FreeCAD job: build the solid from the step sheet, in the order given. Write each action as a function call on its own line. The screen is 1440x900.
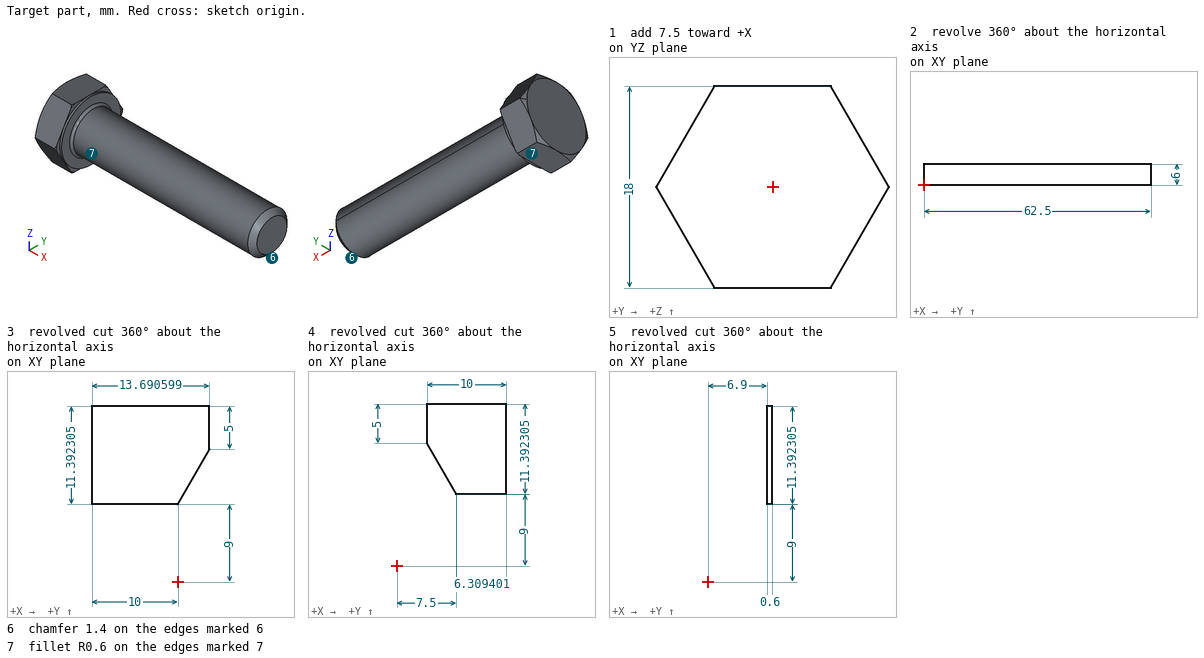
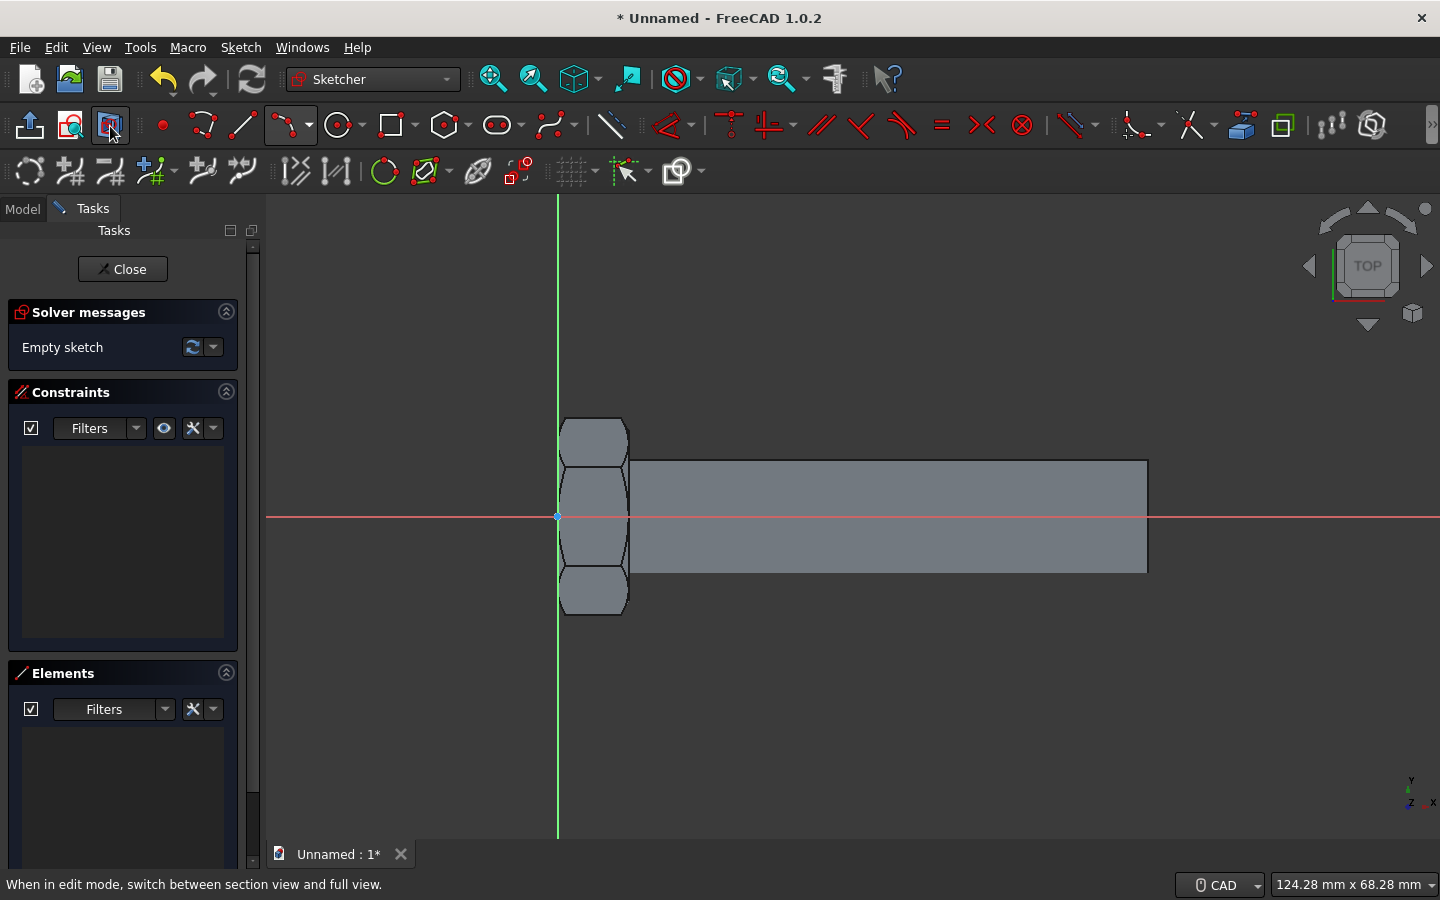
scroll(437, 342, up, 4)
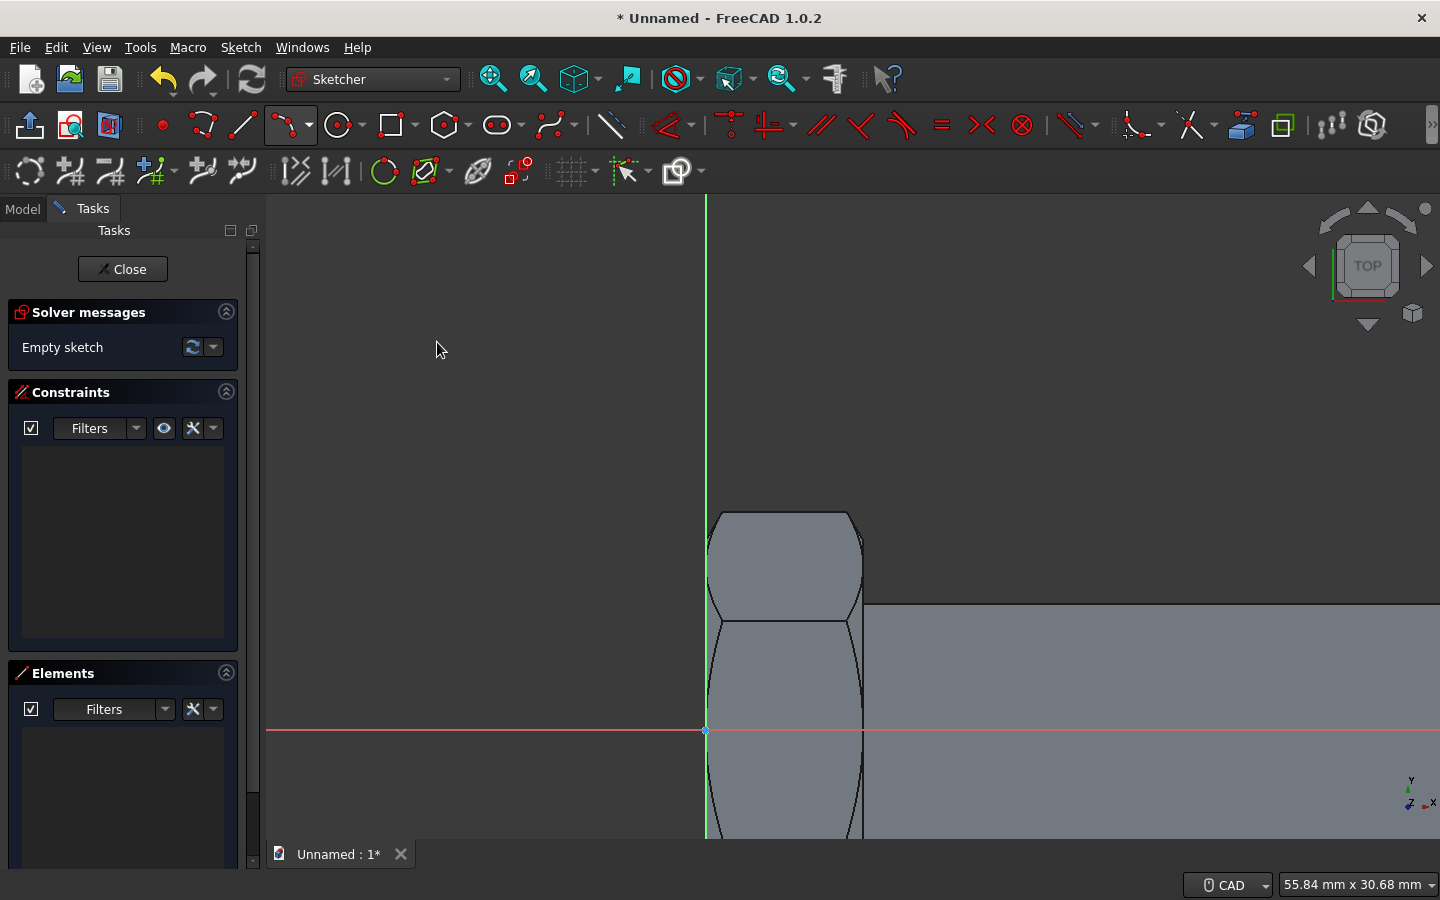
click(392, 126)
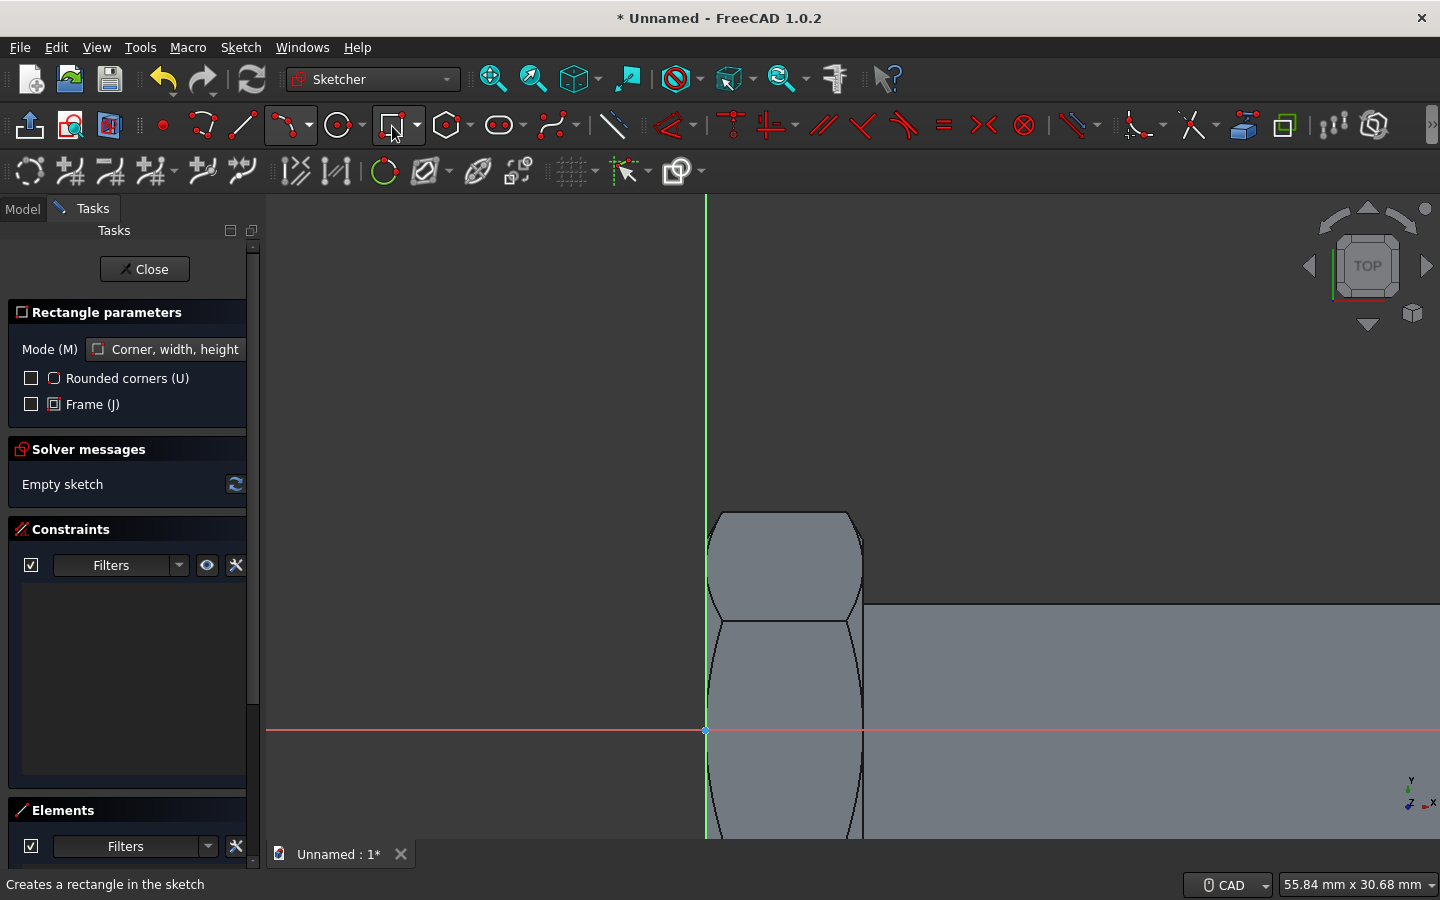
scroll(851, 301, up, 2)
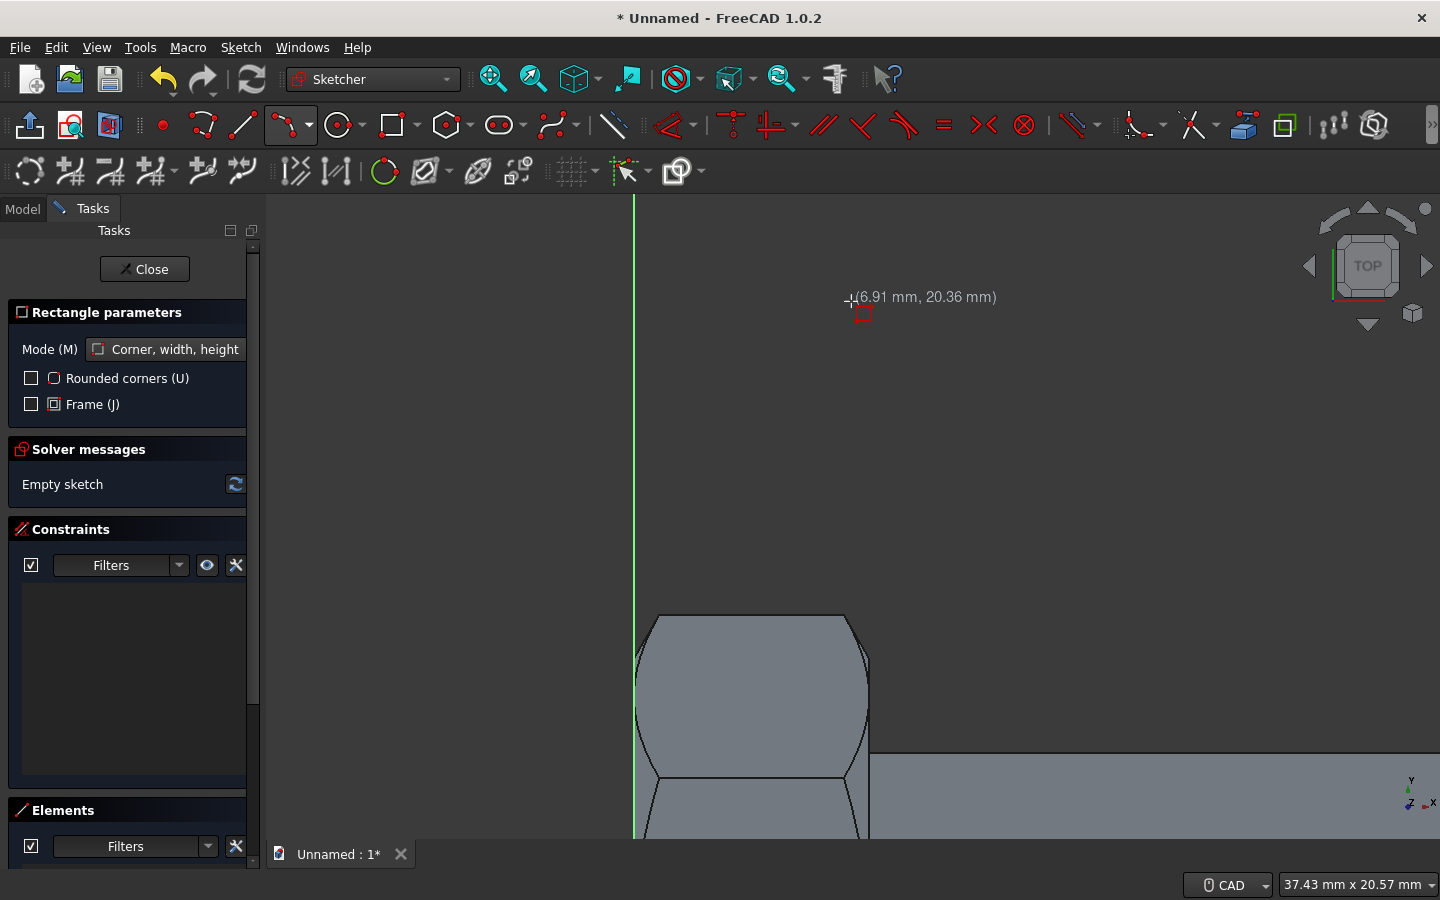
click(850, 301)
click(869, 659)
key(Escape)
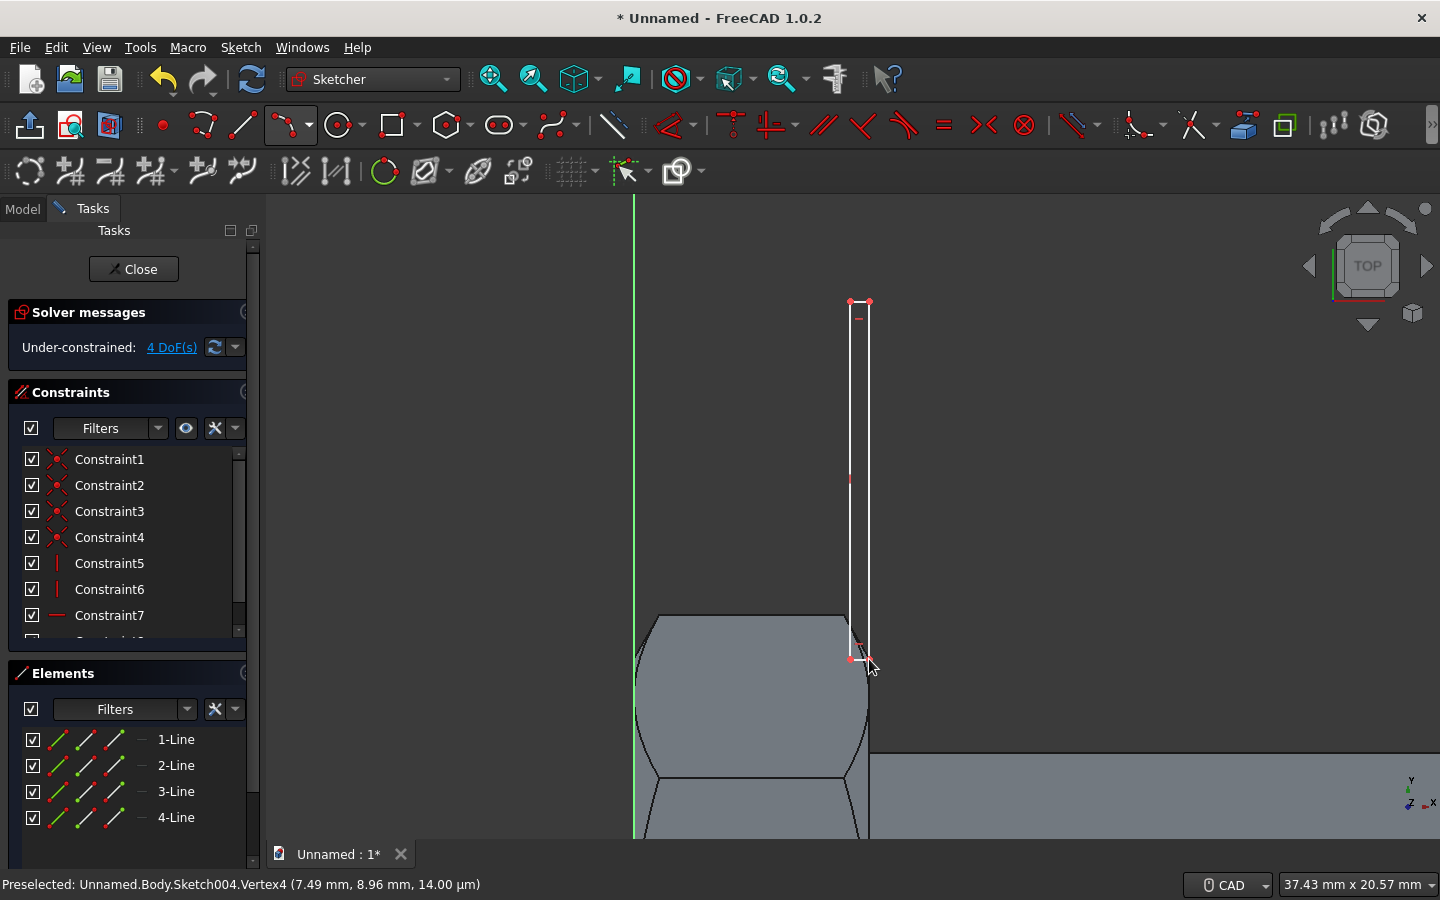
click(668, 126)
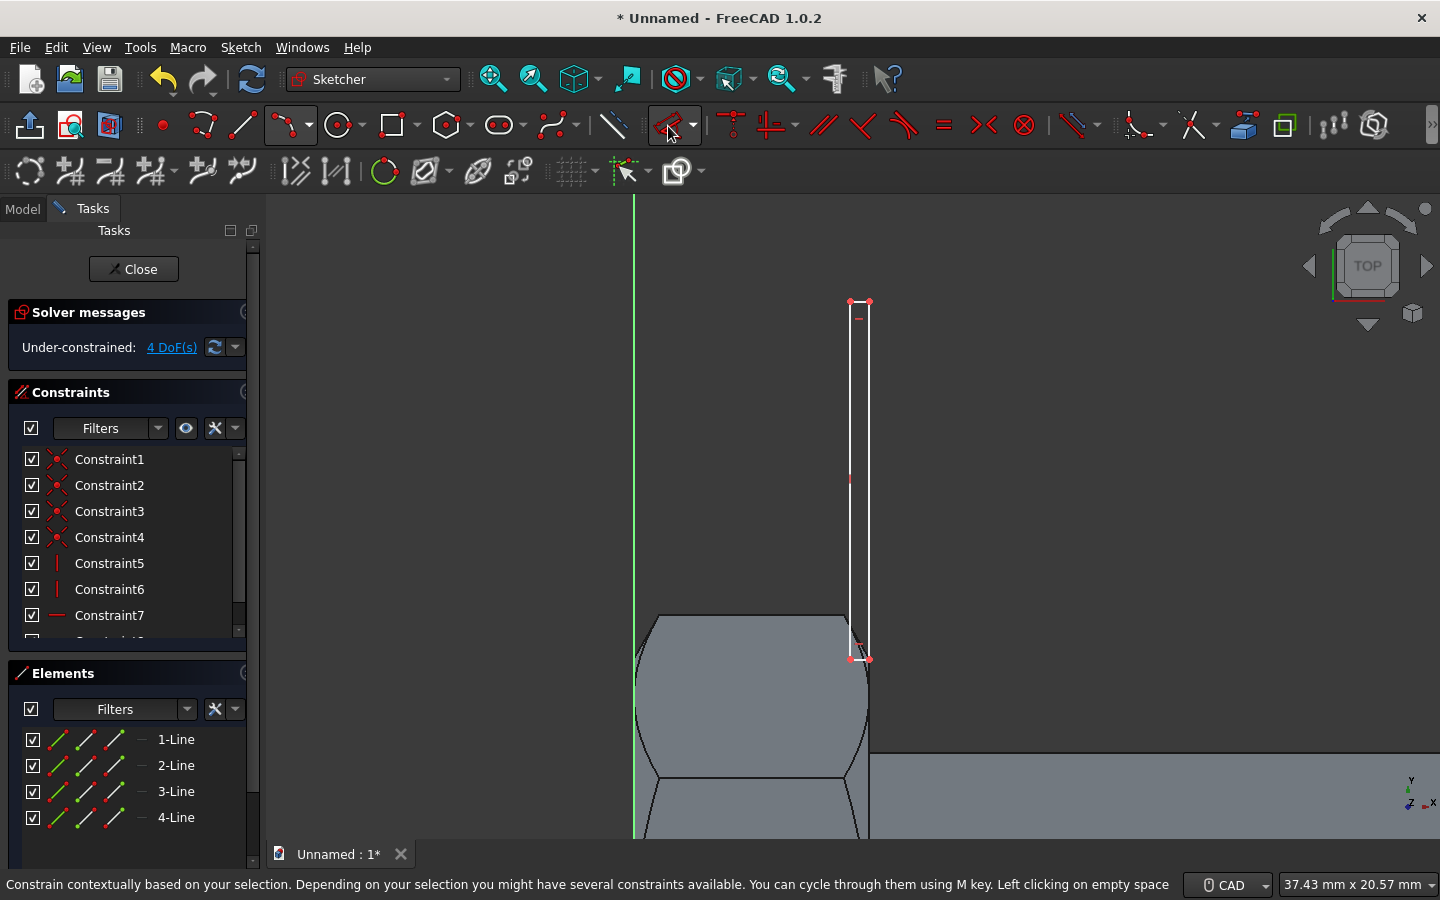
click(850, 660)
click(600, 735)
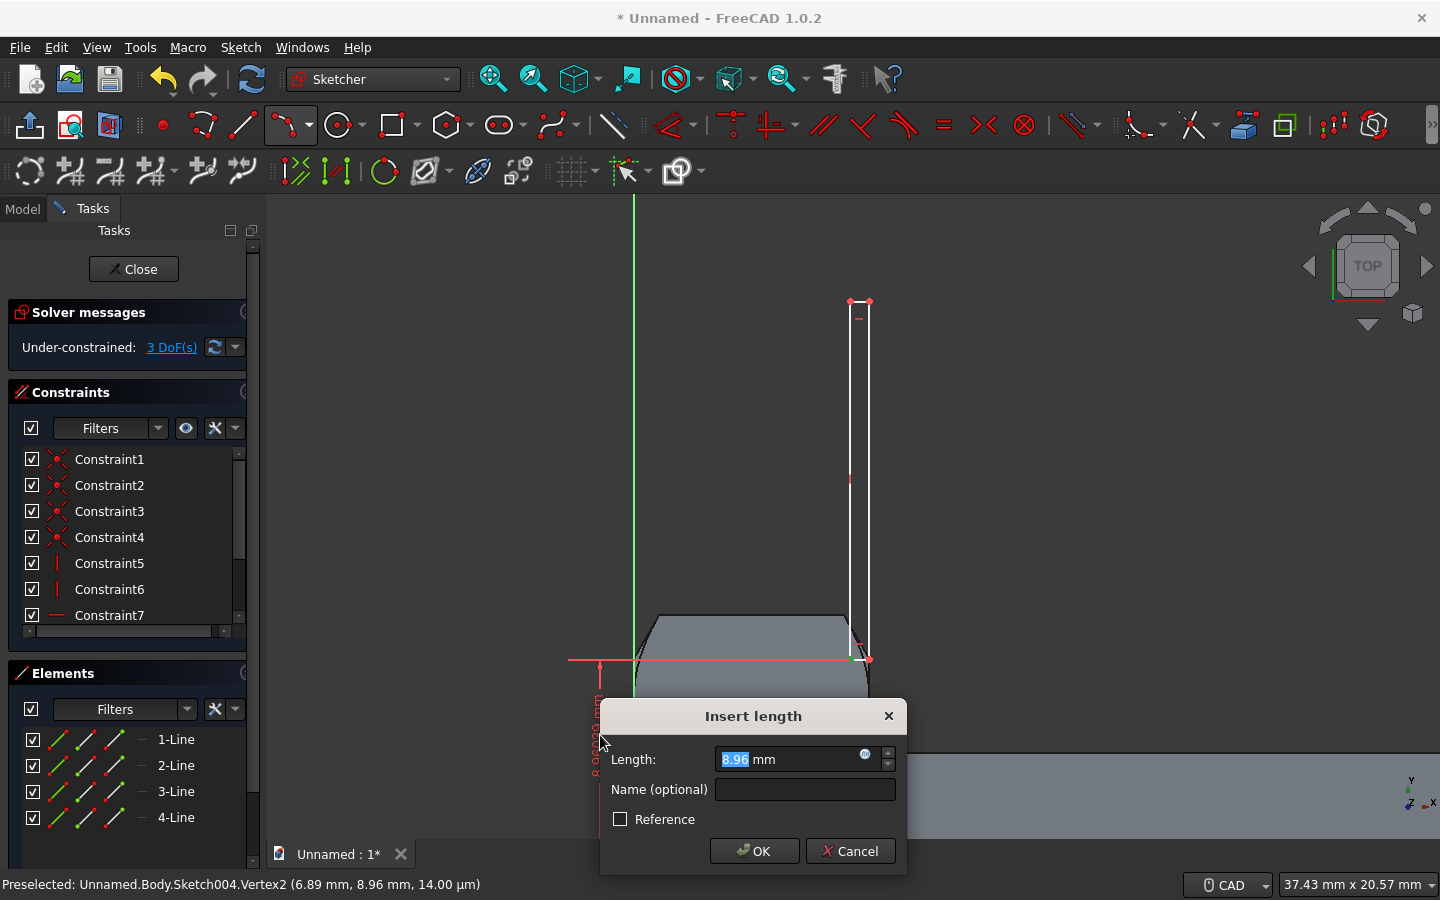
text(9)
key(Return)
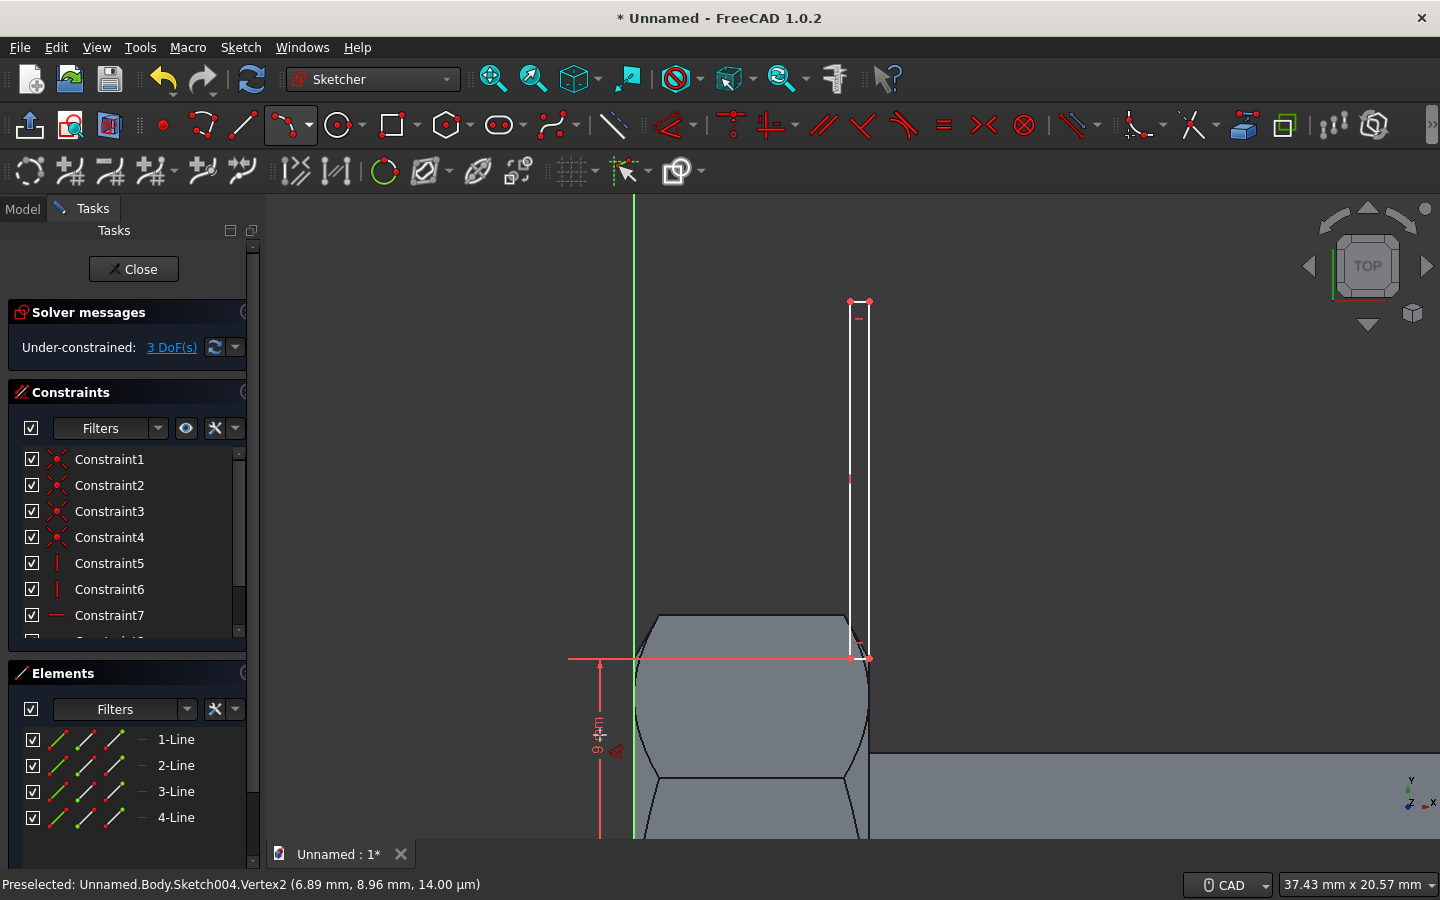
scroll(859, 659, up, 4)